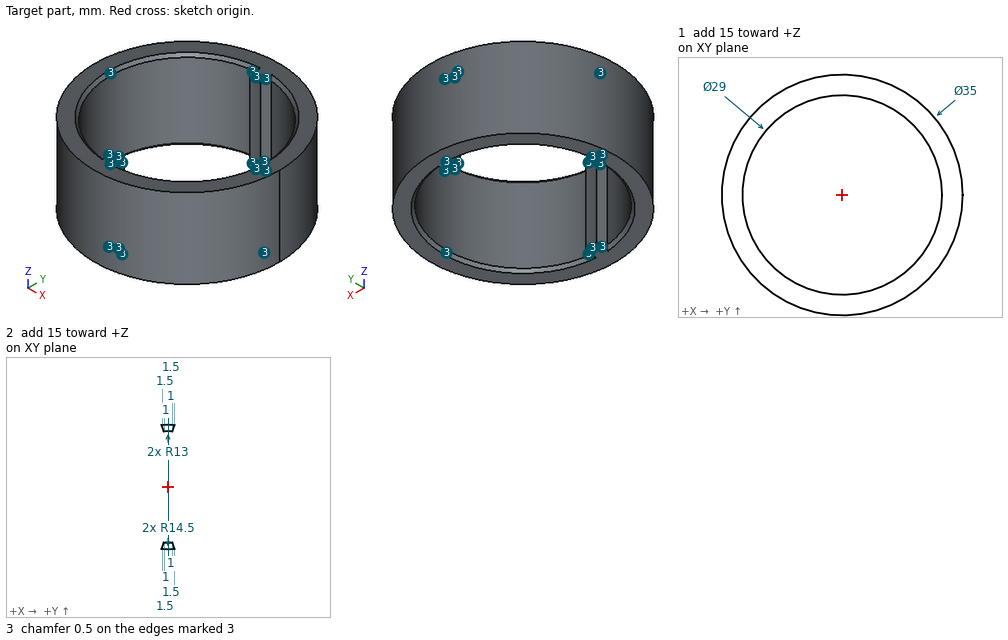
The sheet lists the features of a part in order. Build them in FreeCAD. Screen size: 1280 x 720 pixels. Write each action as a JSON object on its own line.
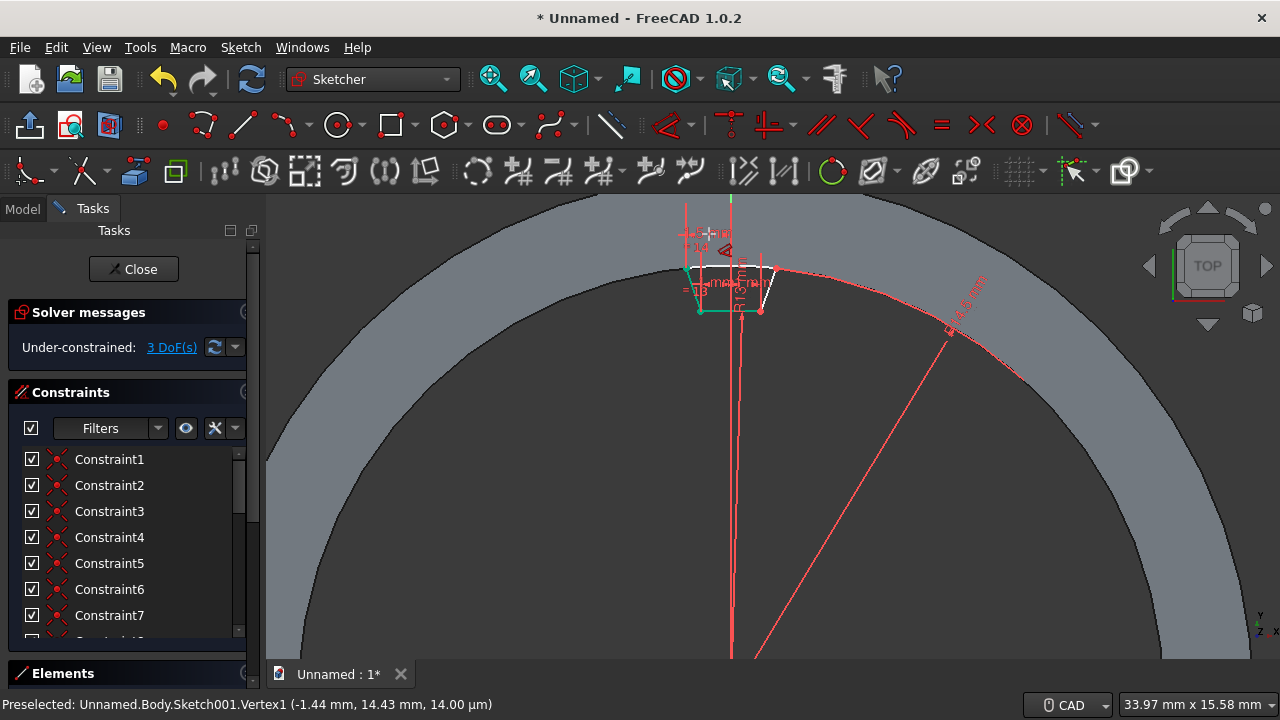
{"action": "left_click", "coordinate": [776, 268]}
{"action": "left_click", "coordinate": [754, 234]}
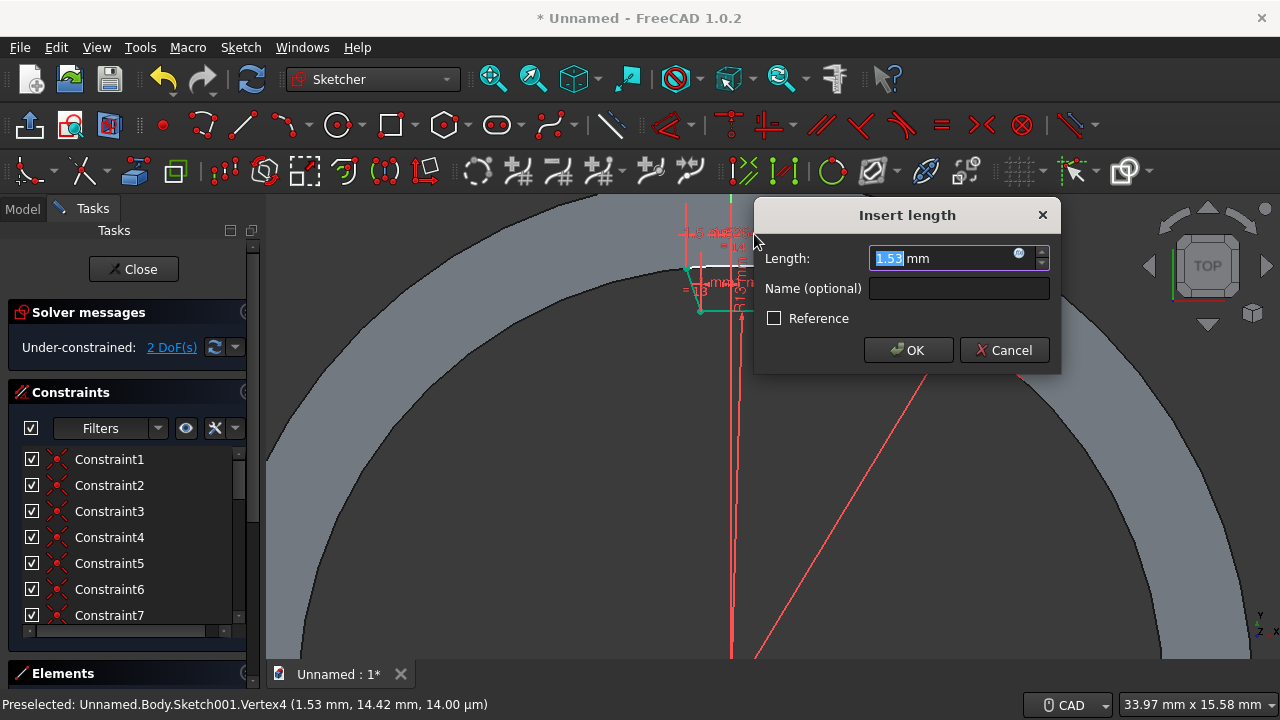
{"action": "type", "text": "1.5"}
{"action": "key", "text": "Return"}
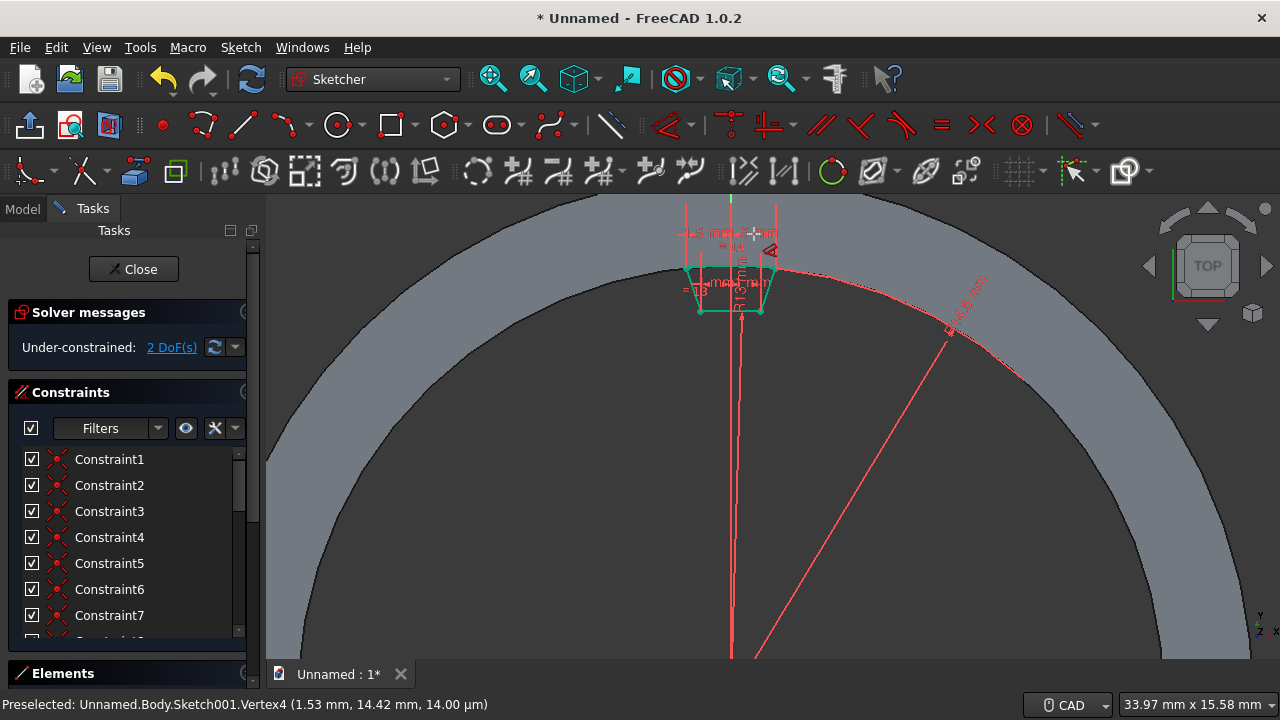
{"action": "scroll", "coordinate": [689, 268], "scroll_direction": "down", "scroll_amount": 5}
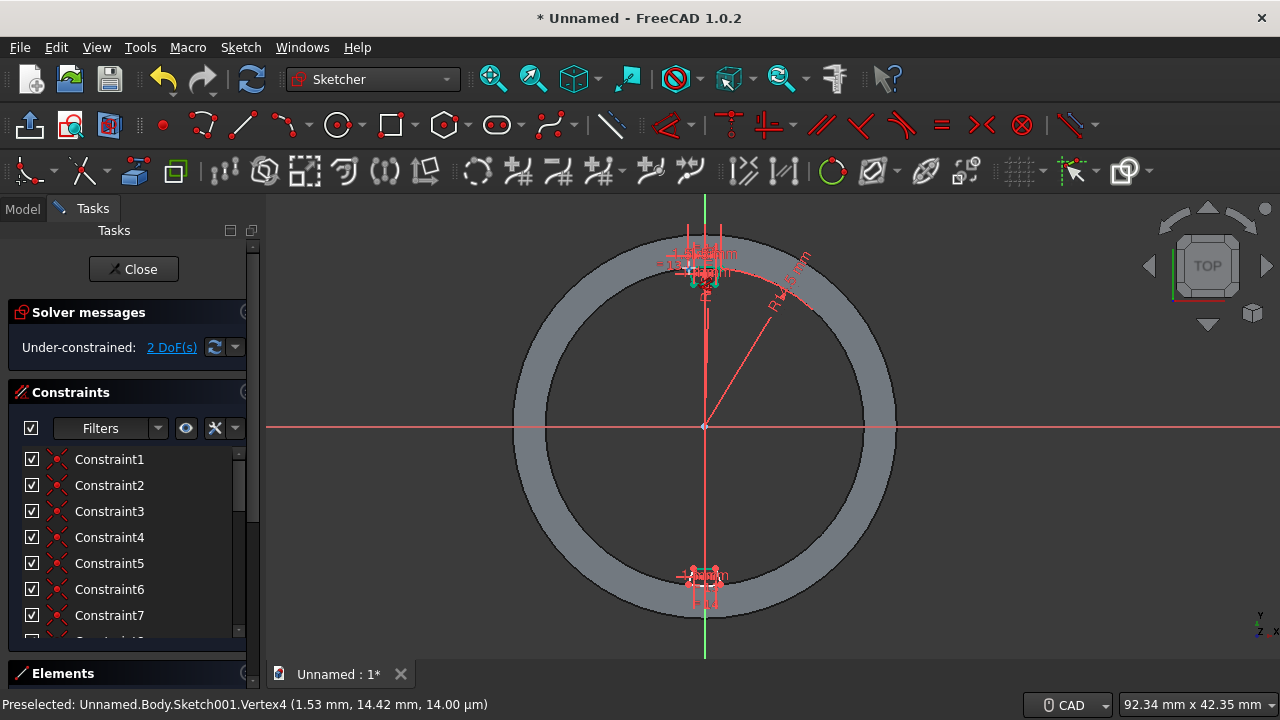
{"action": "scroll", "coordinate": [721, 585], "scroll_direction": "up", "scroll_amount": 5}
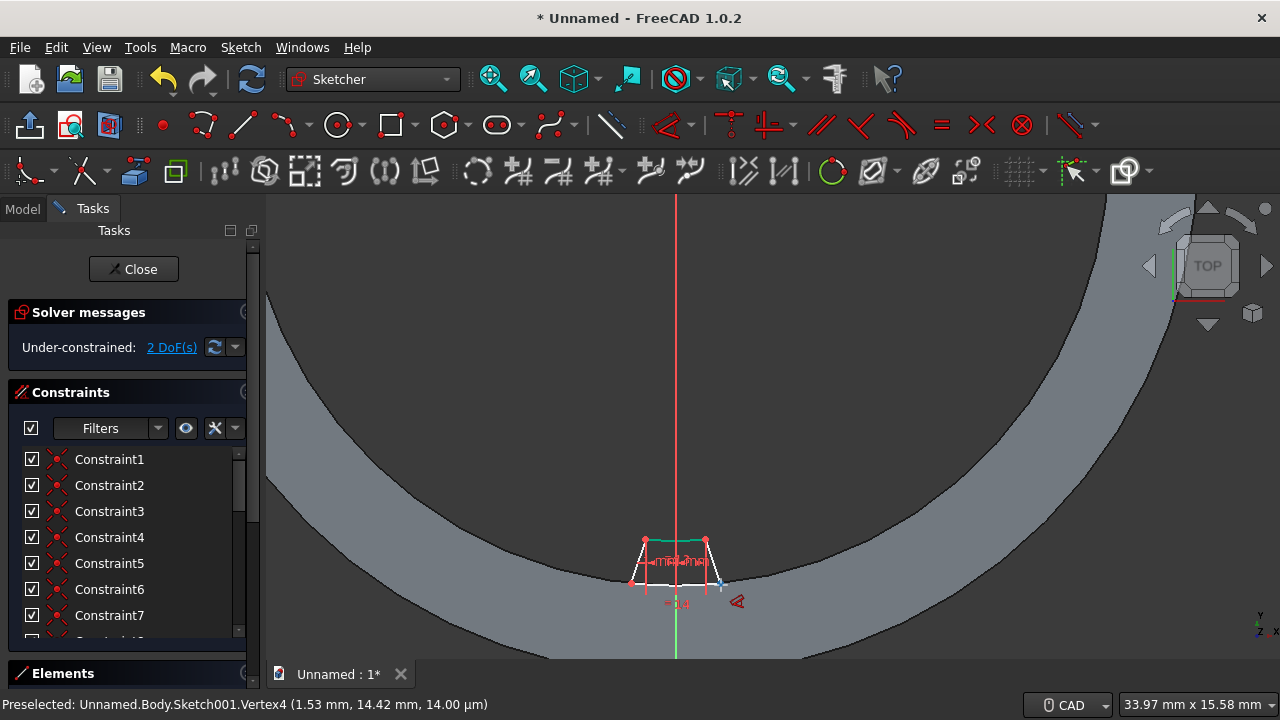
{"action": "left_click", "coordinate": [720, 583]}
{"action": "left_click", "coordinate": [698, 617]}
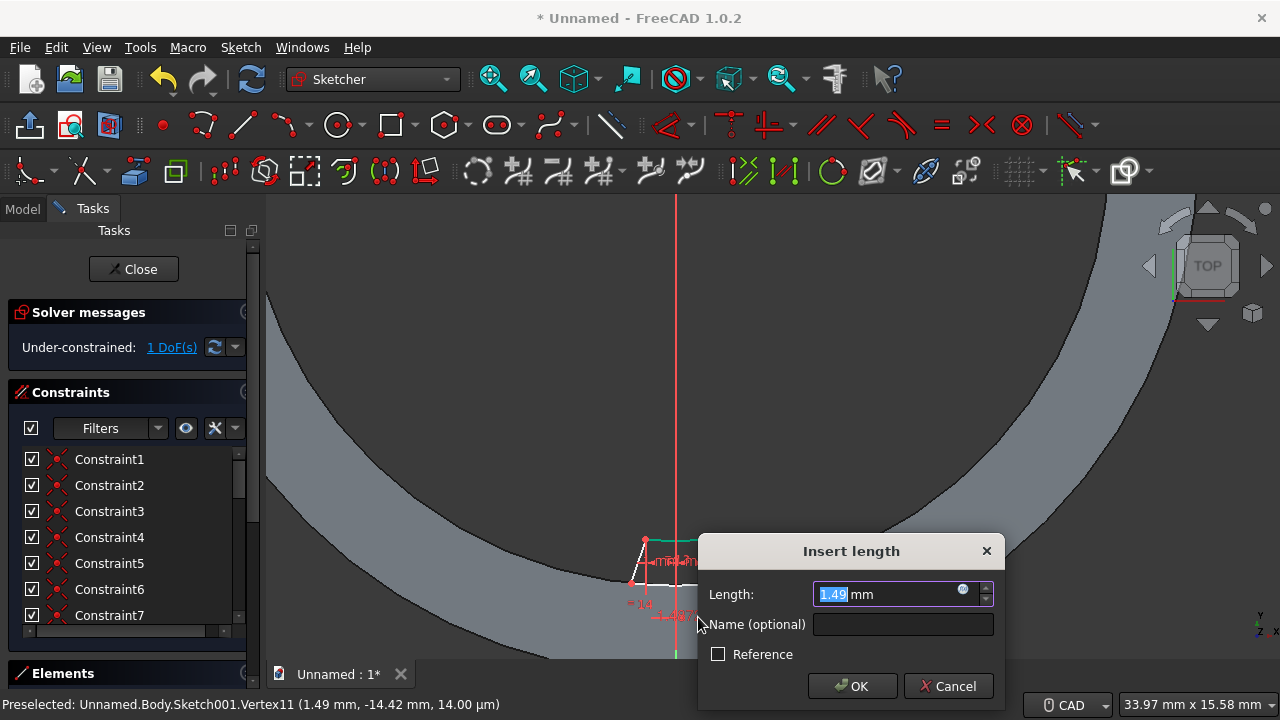
{"action": "type", "text": "1.5"}
{"action": "key", "text": "Return"}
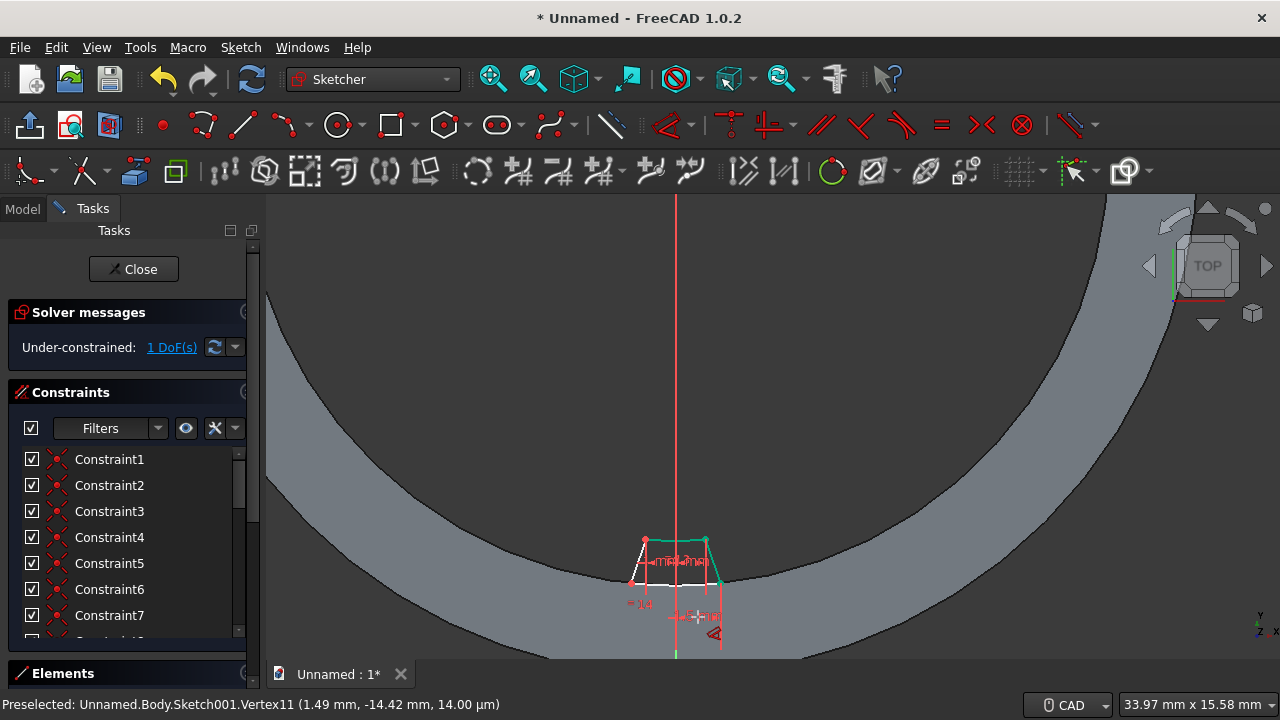
{"action": "left_click", "coordinate": [631, 583]}
{"action": "left_click", "coordinate": [653, 617]}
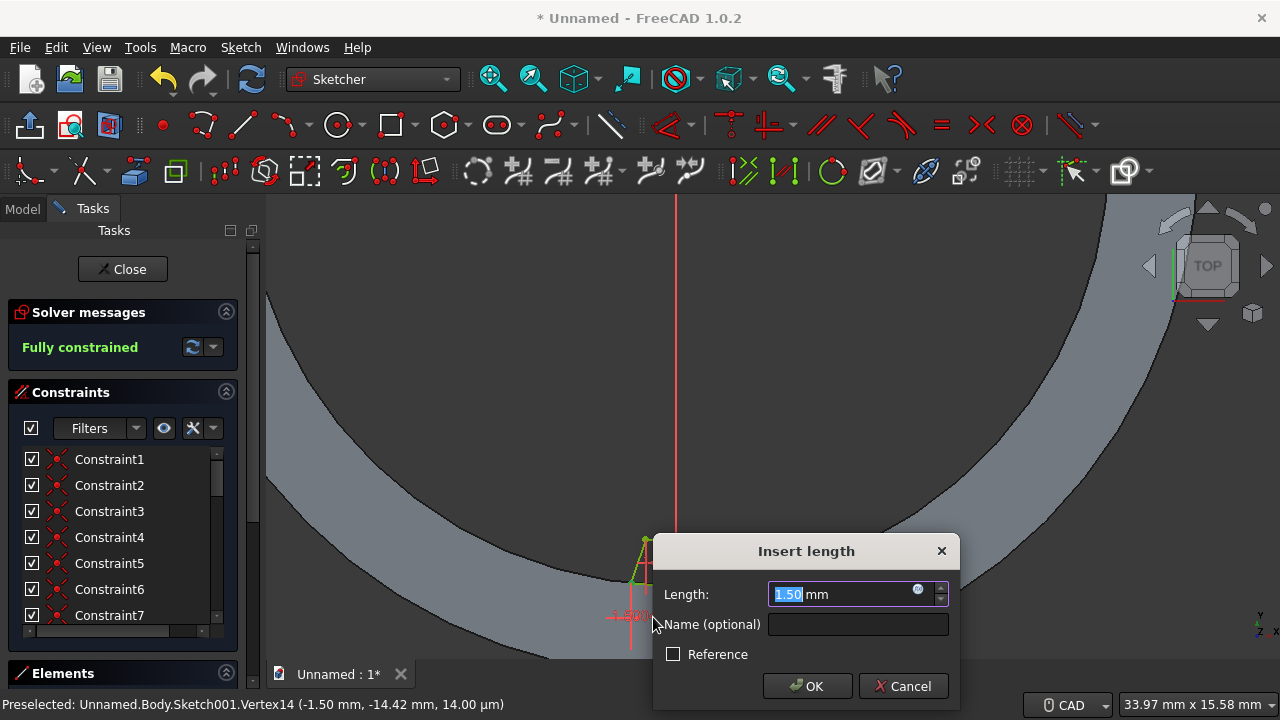
{"action": "type", "text": "1.5"}
{"action": "key", "text": "Return"}
{"action": "key", "text": "Escape"}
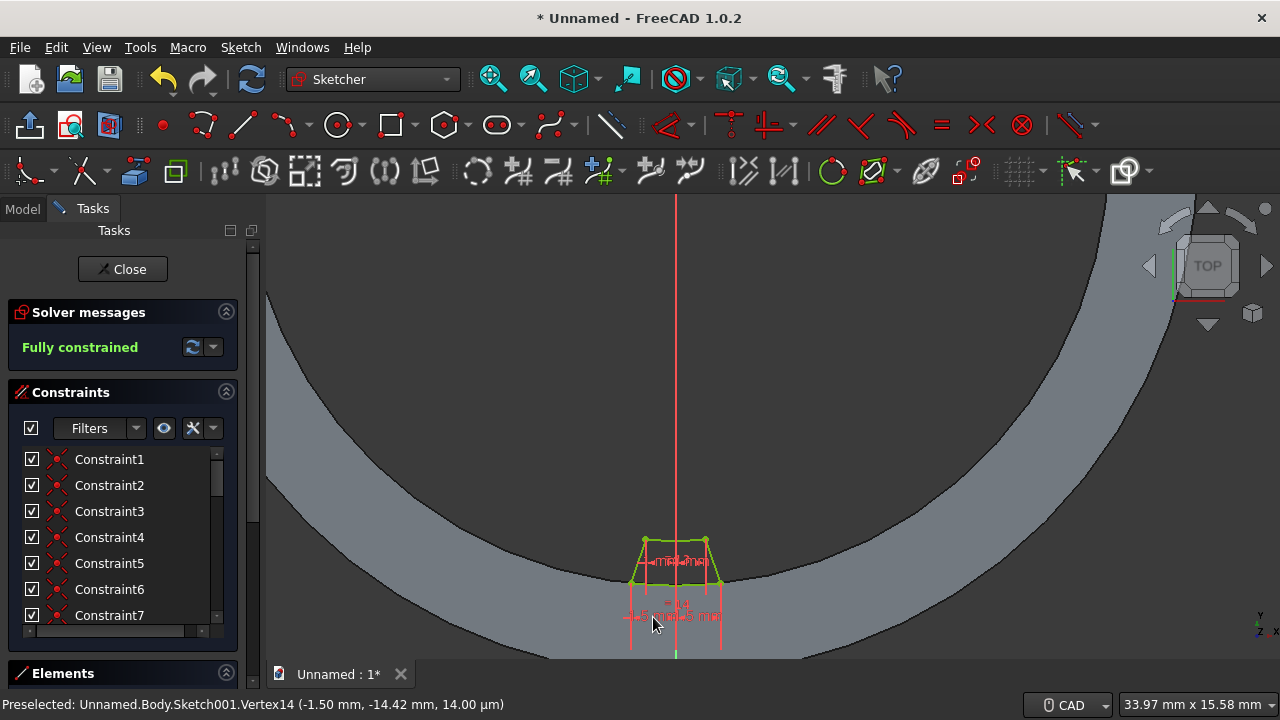
{"action": "left_click", "coordinate": [123, 269]}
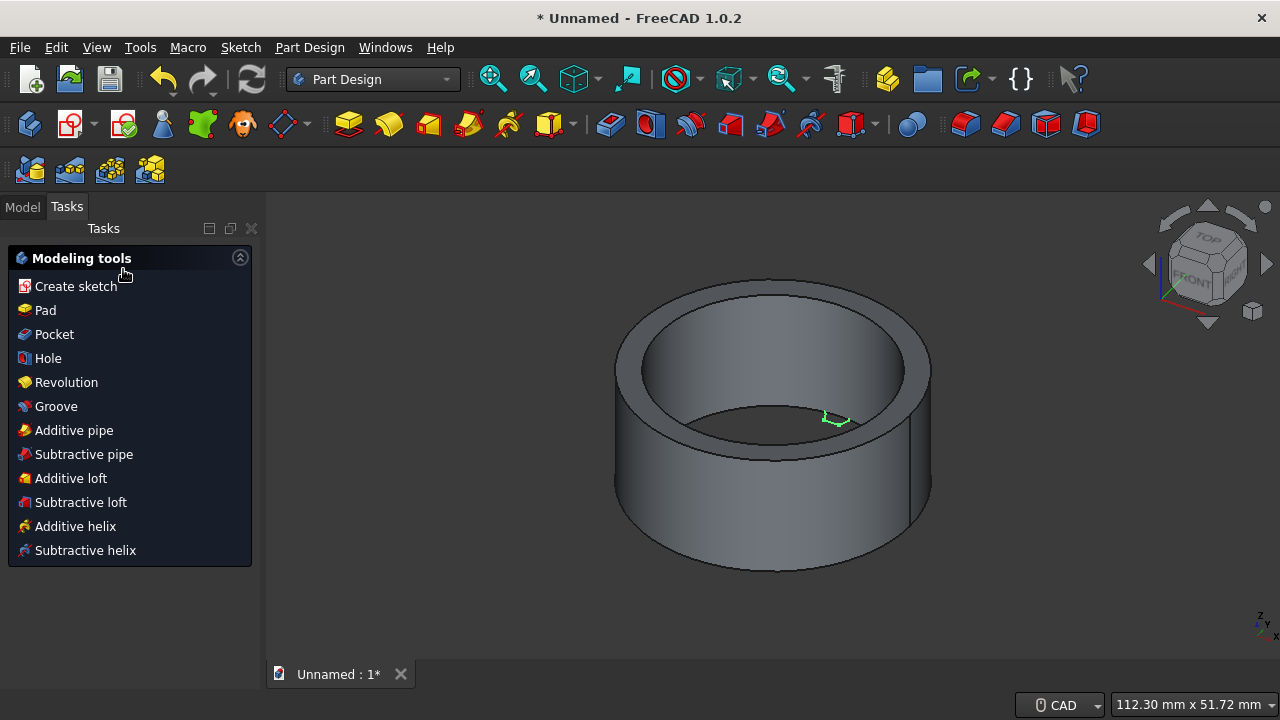
{"action": "left_click", "coordinate": [350, 124]}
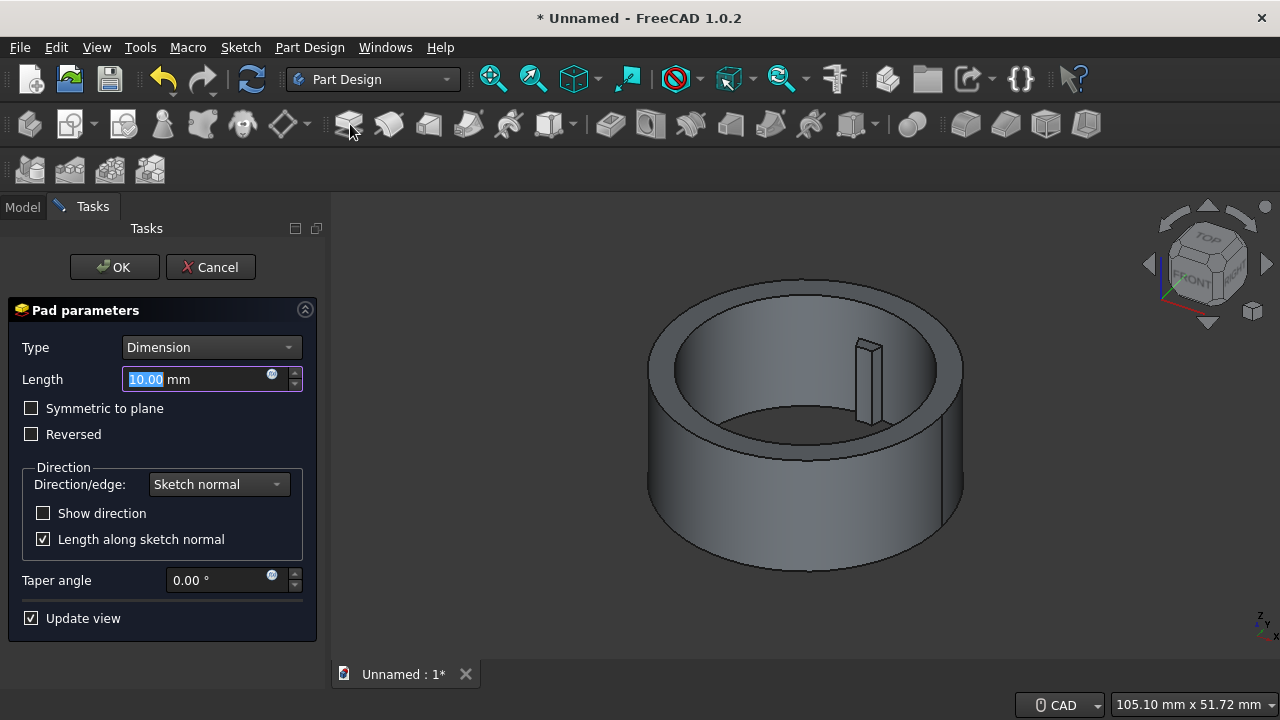
{"action": "type", "text": "15"}
{"action": "key", "text": "Tab"}